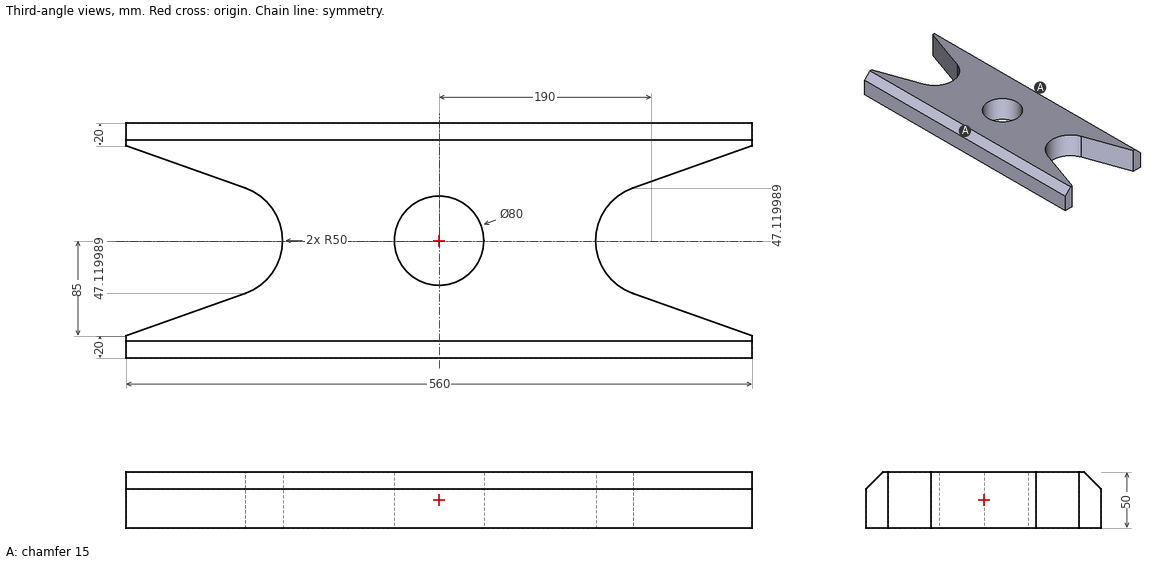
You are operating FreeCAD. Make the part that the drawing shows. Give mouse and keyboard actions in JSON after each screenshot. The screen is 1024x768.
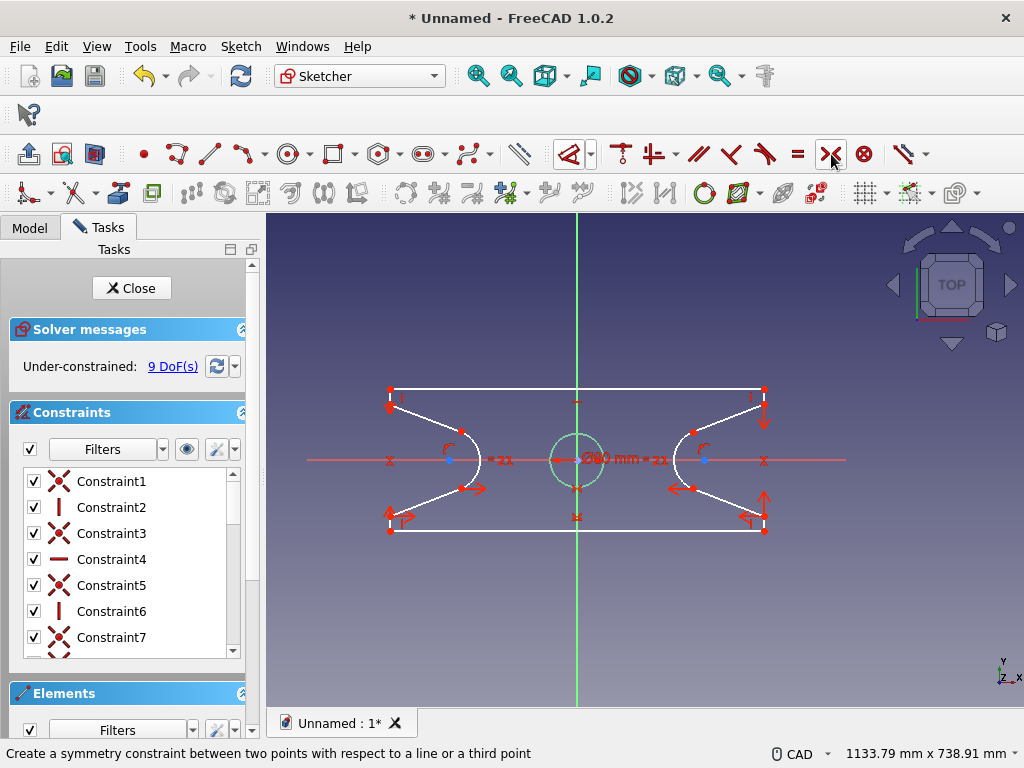
{"action": "left_click", "coordinate": [568, 154]}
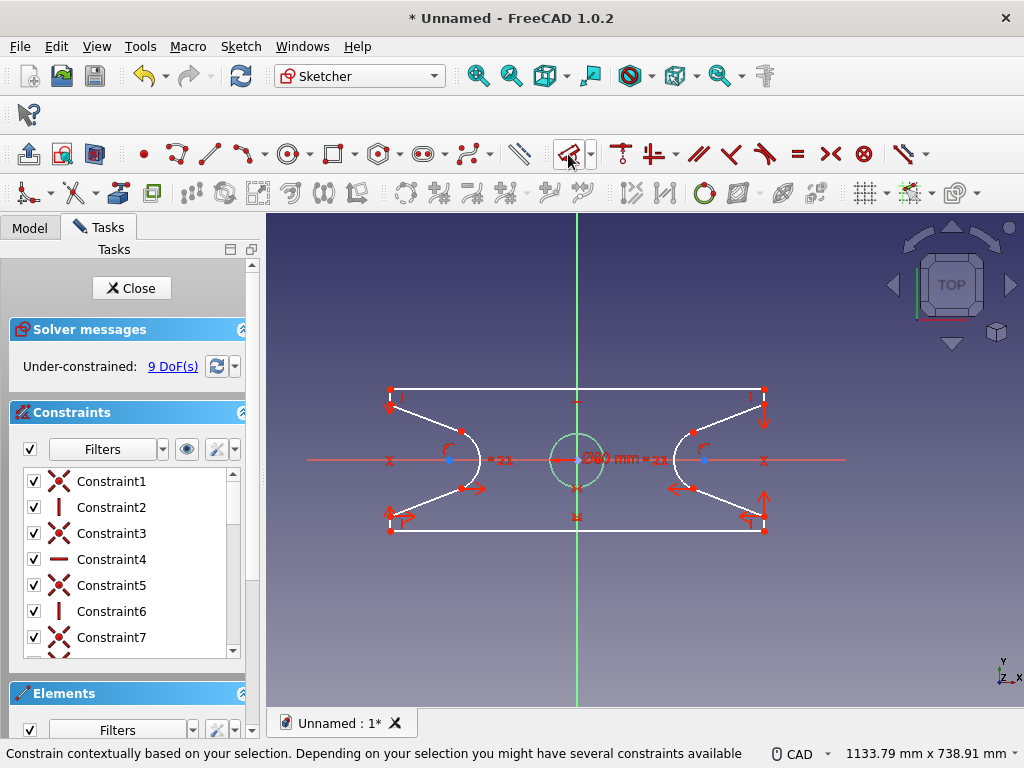
{"action": "left_click", "coordinate": [677, 446]}
{"action": "left_click", "coordinate": [649, 431]}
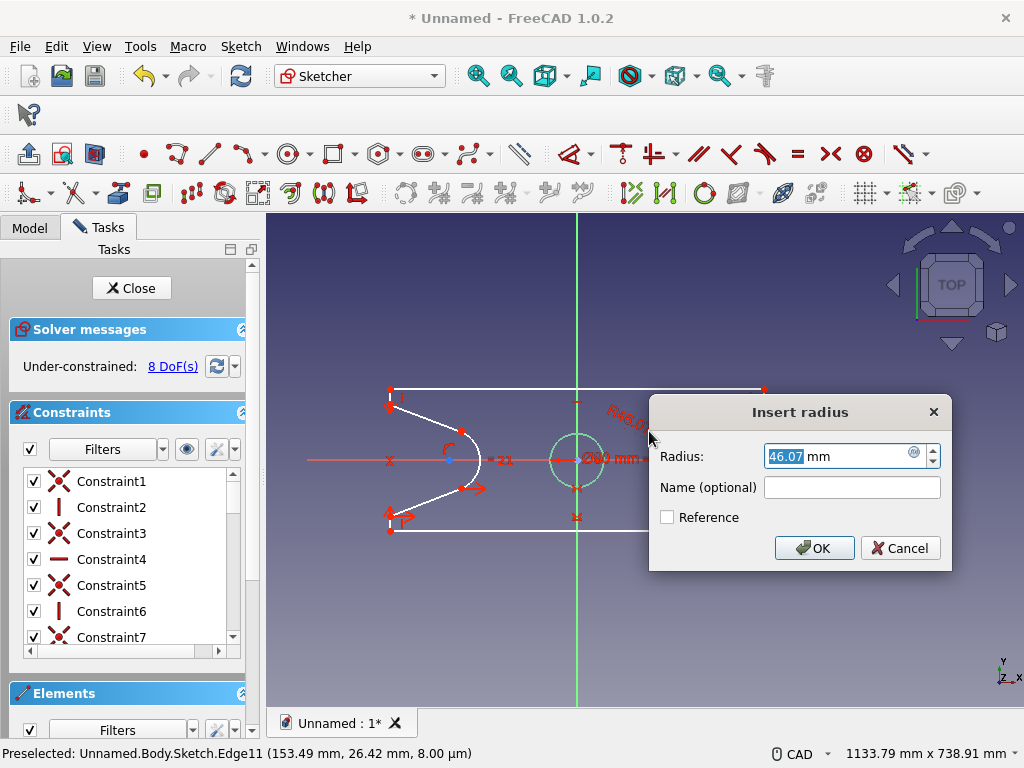
{"action": "type", "text": "50"}
{"action": "key", "text": "Return"}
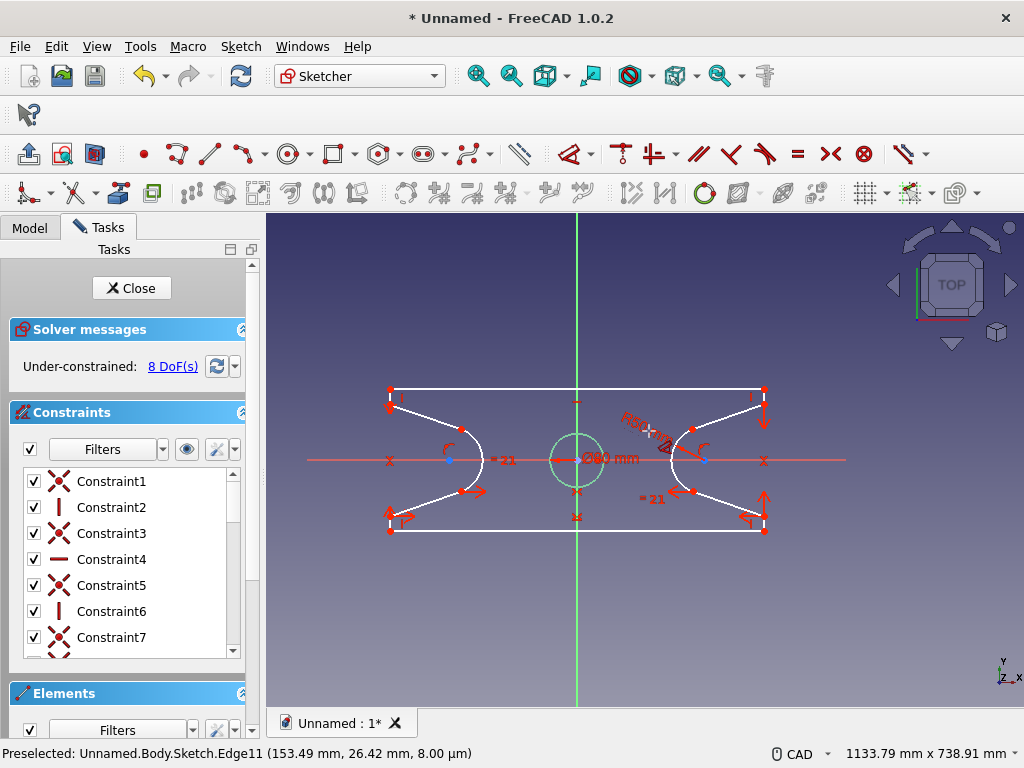
{"action": "scroll", "coordinate": [390, 524], "scroll_direction": "up", "scroll_amount": 6}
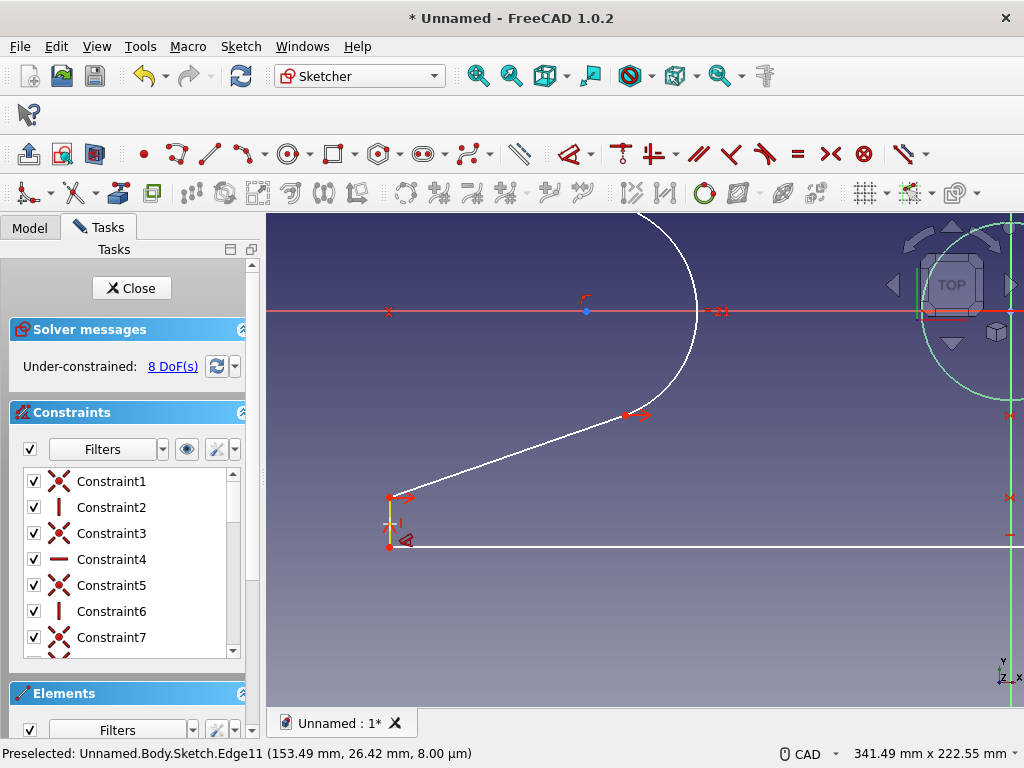
{"action": "left_click", "coordinate": [390, 522]}
{"action": "left_click", "coordinate": [356, 522]}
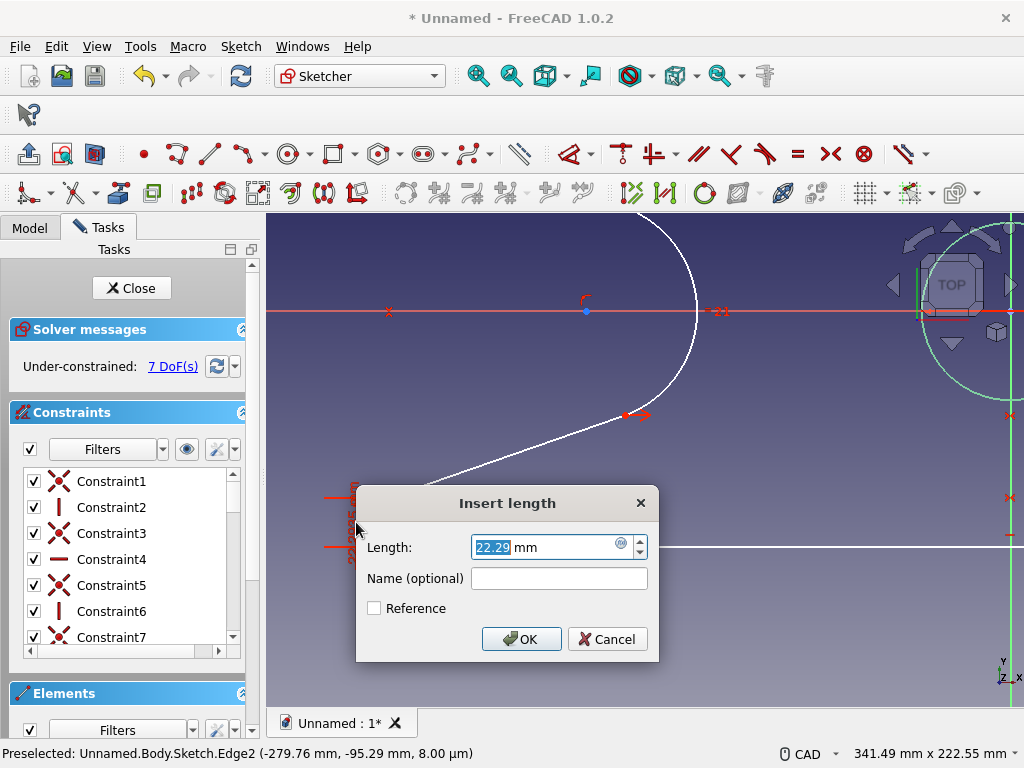
{"action": "type", "text": "20"}
{"action": "key", "text": "Return"}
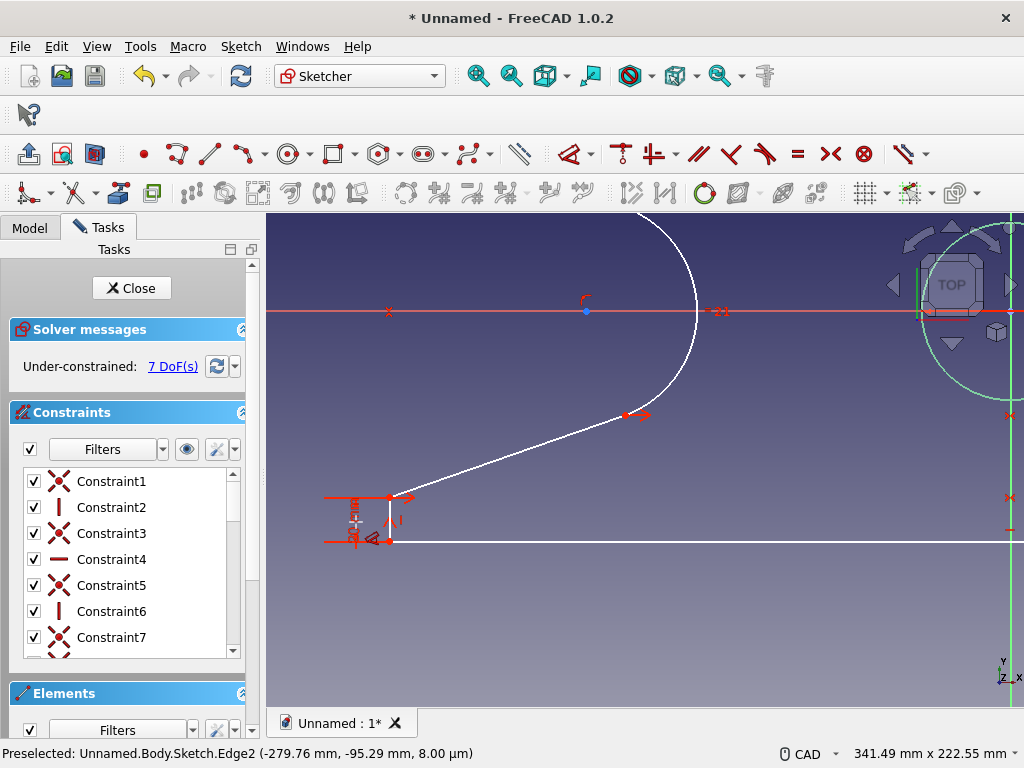
{"action": "scroll", "coordinate": [389, 524], "scroll_direction": "down", "scroll_amount": 6}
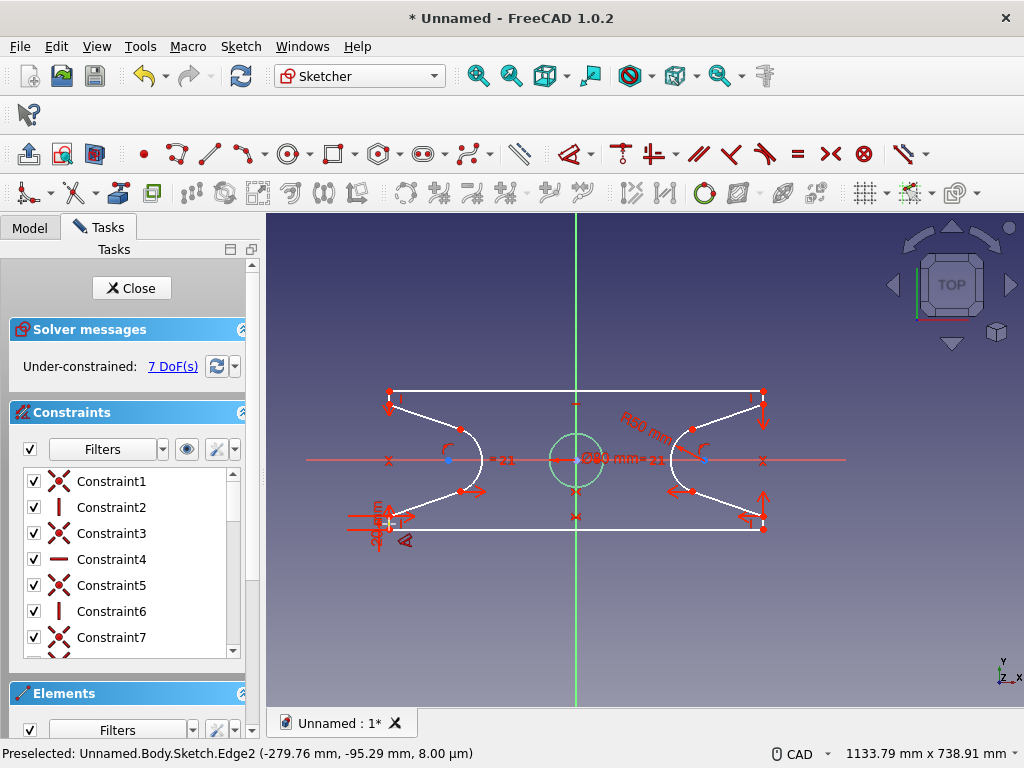
{"action": "scroll", "coordinate": [389, 395], "scroll_direction": "up", "scroll_amount": 6}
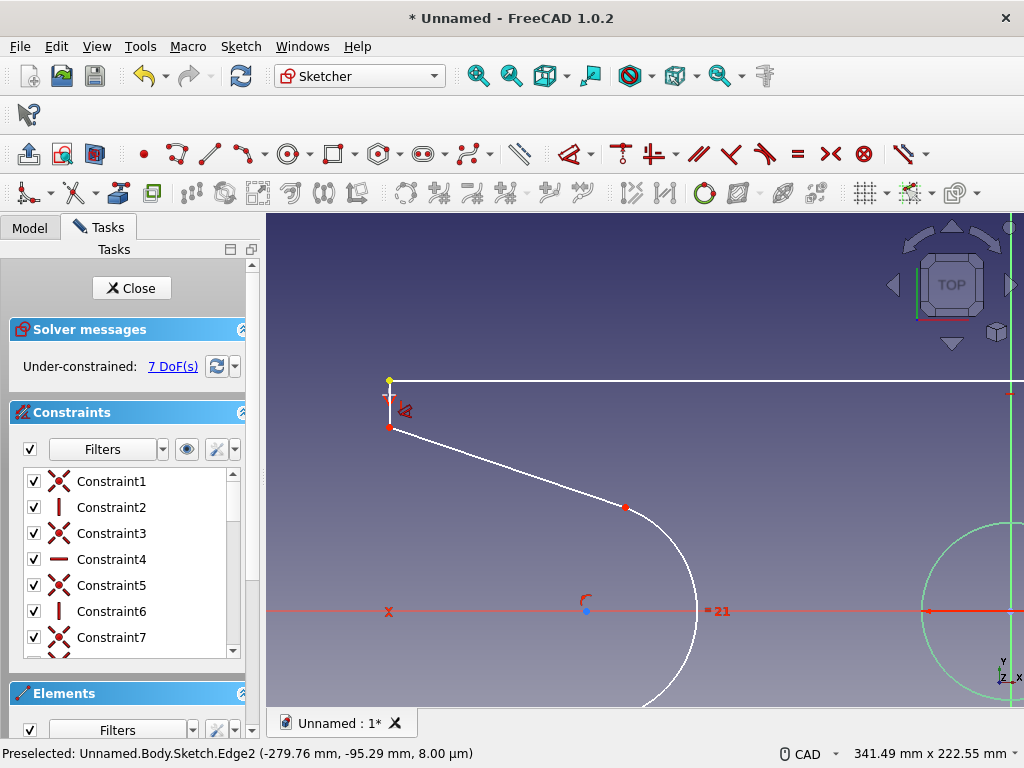
{"action": "left_click", "coordinate": [390, 395]}
{"action": "left_click", "coordinate": [356, 404]}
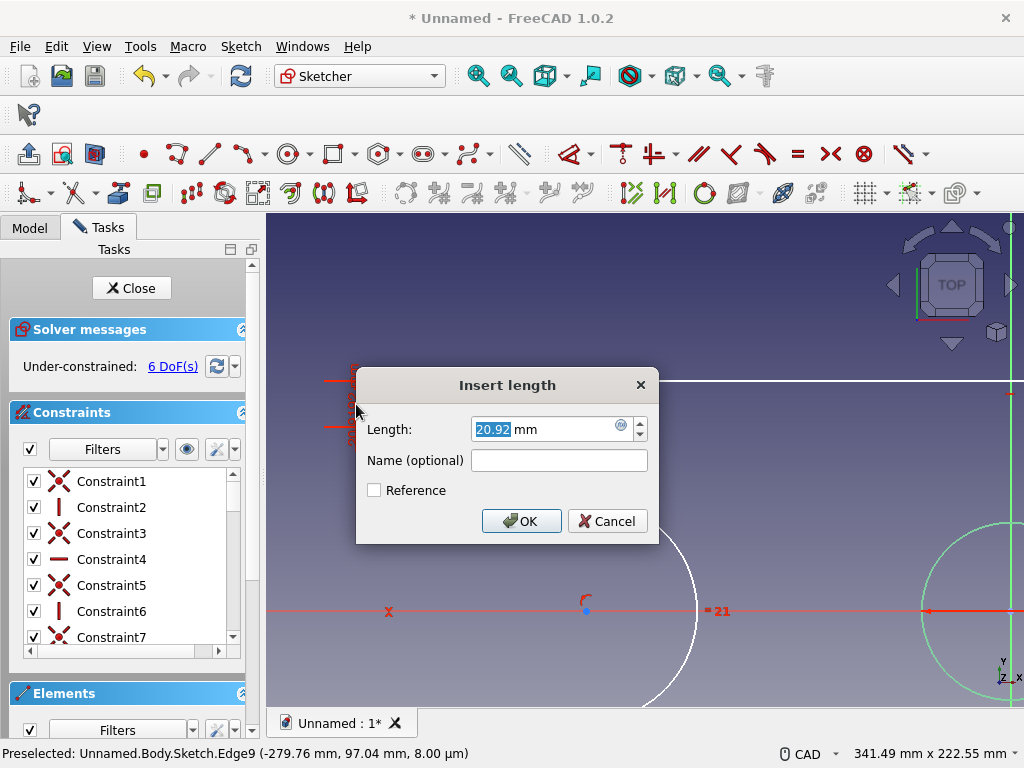
{"action": "type", "text": "20"}
{"action": "key", "text": "Return"}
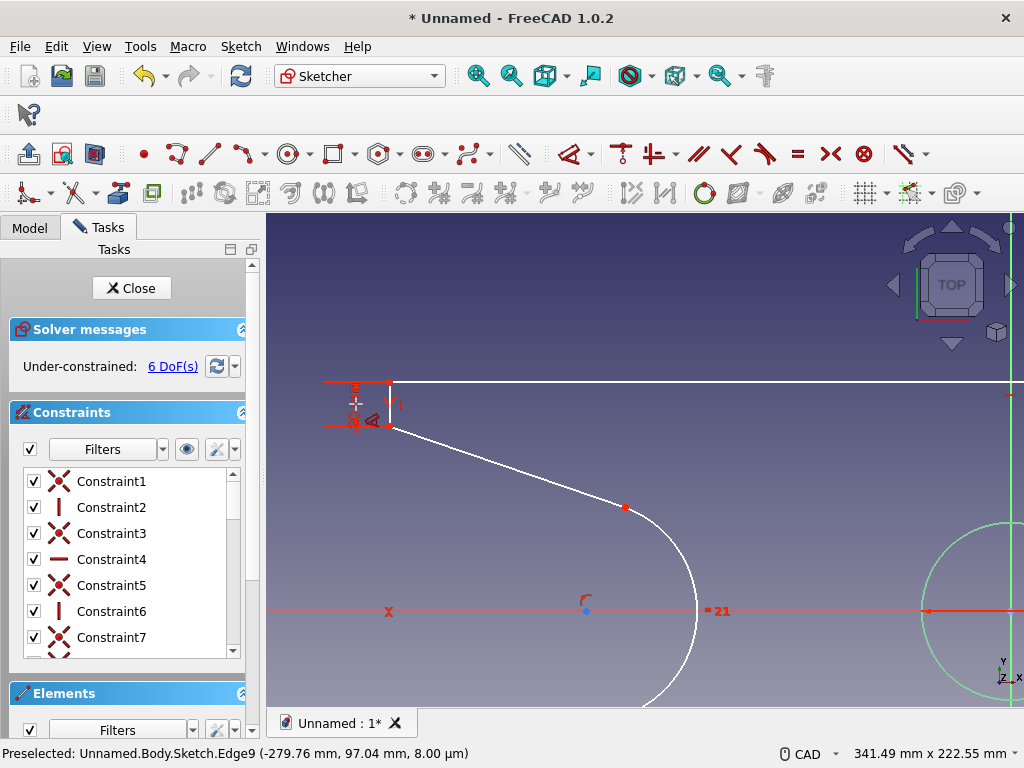
{"action": "scroll", "coordinate": [389, 395], "scroll_direction": "down", "scroll_amount": 6}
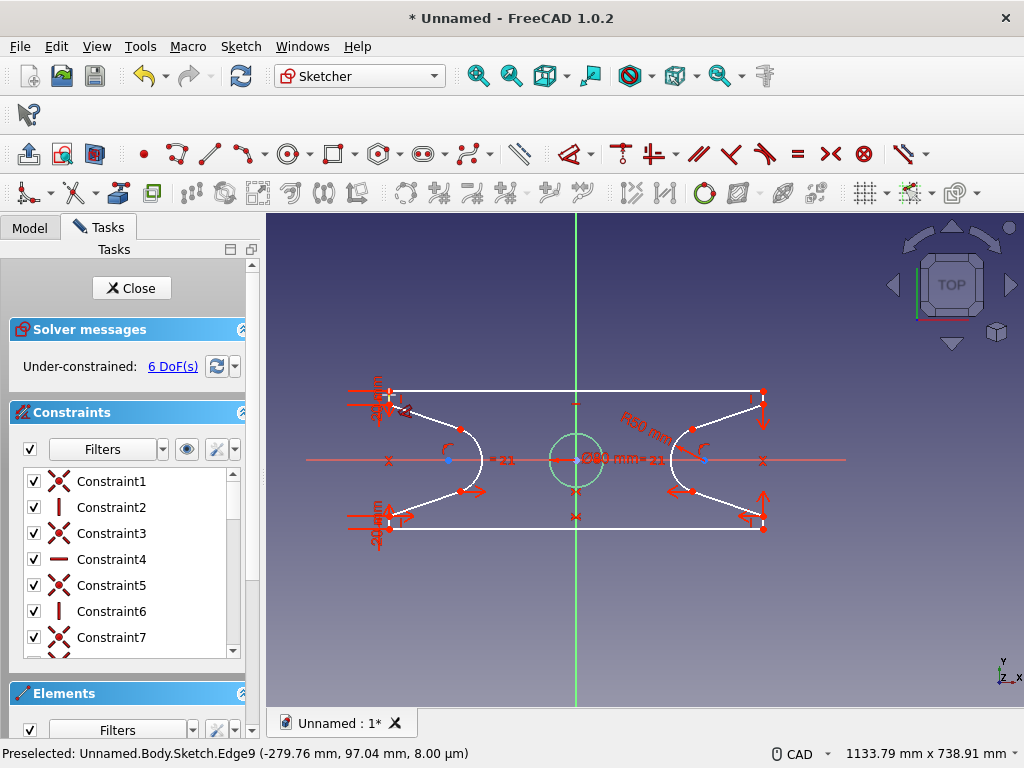
{"action": "left_click", "coordinate": [502, 529]}
{"action": "left_click", "coordinate": [490, 563]}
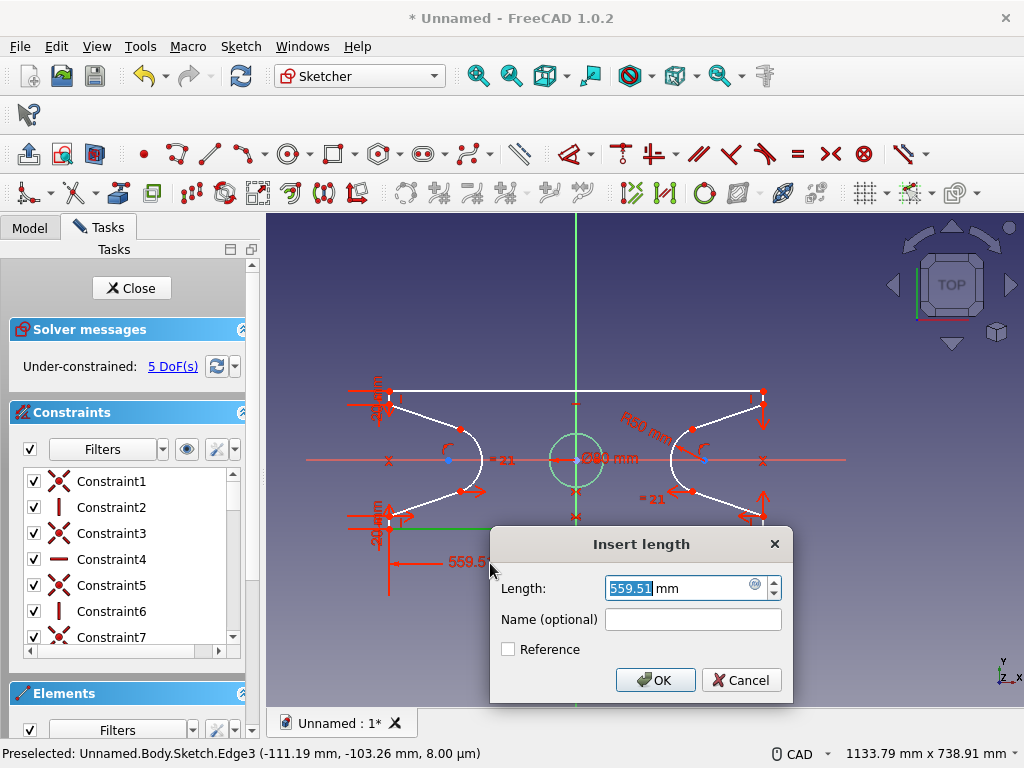
{"action": "type", "text": "560"}
{"action": "key", "text": "Return"}